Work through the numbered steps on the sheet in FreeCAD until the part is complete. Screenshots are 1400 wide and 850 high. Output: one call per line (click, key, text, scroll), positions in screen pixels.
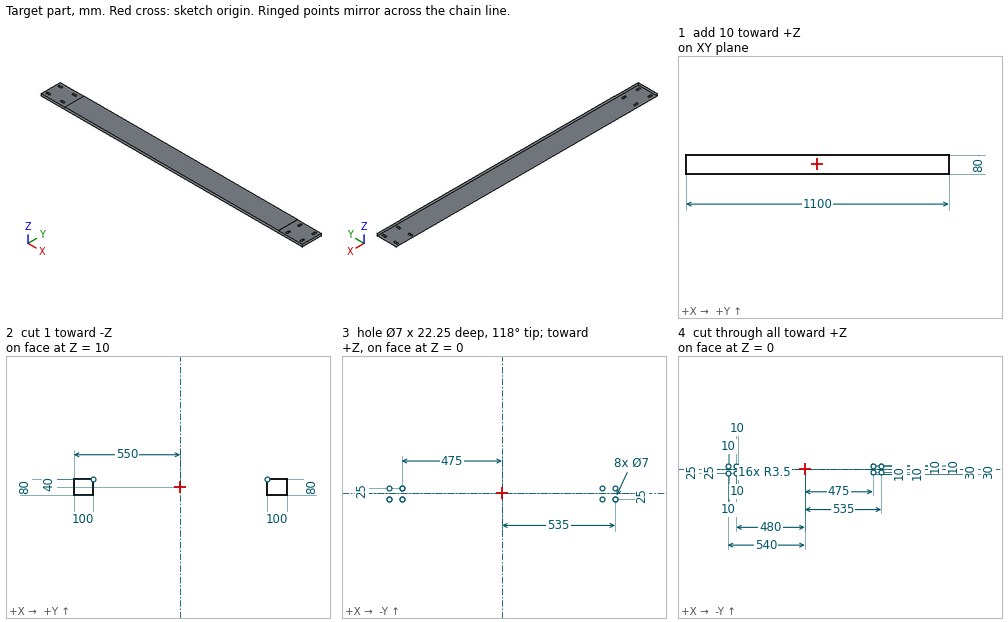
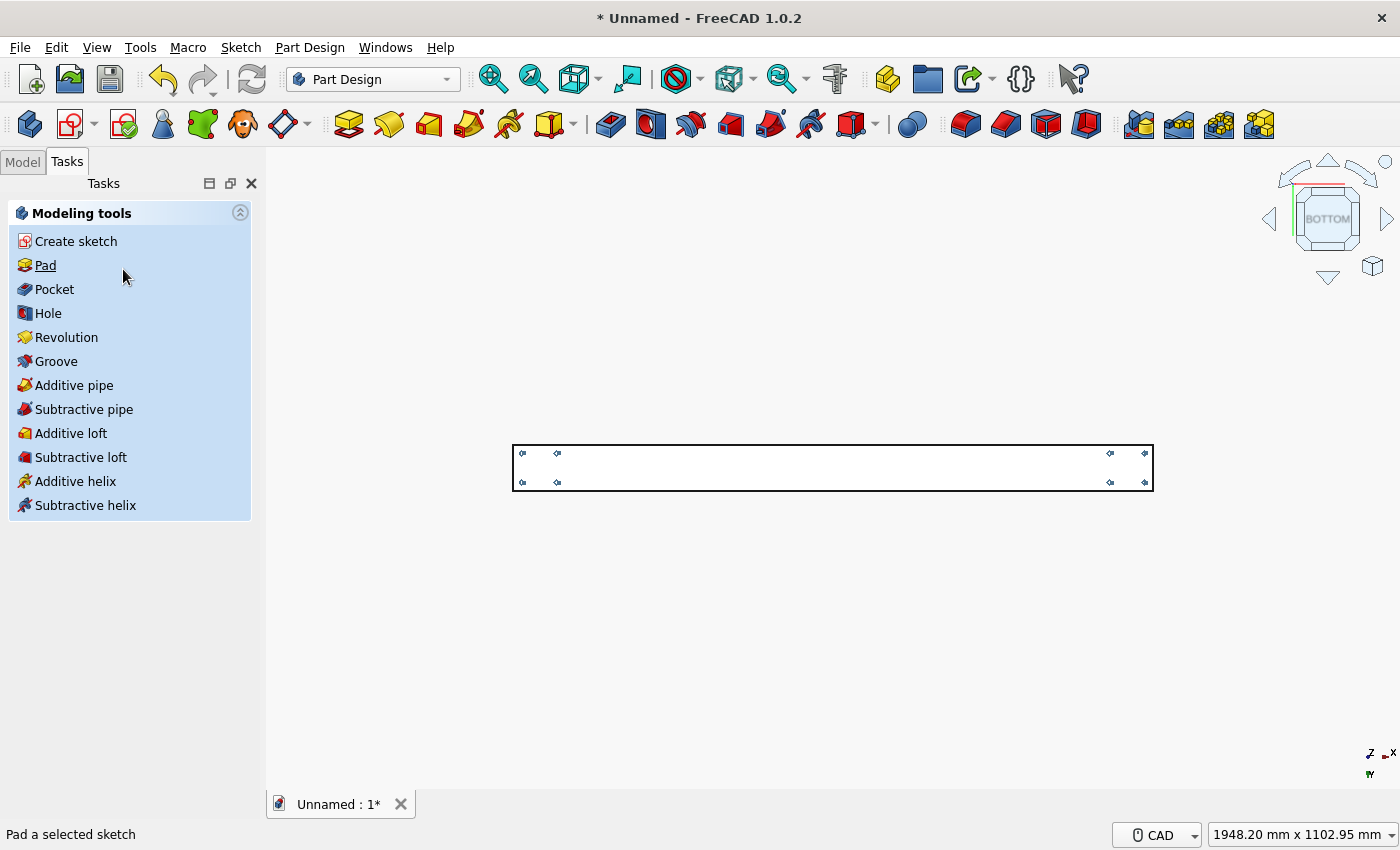
click(652, 124)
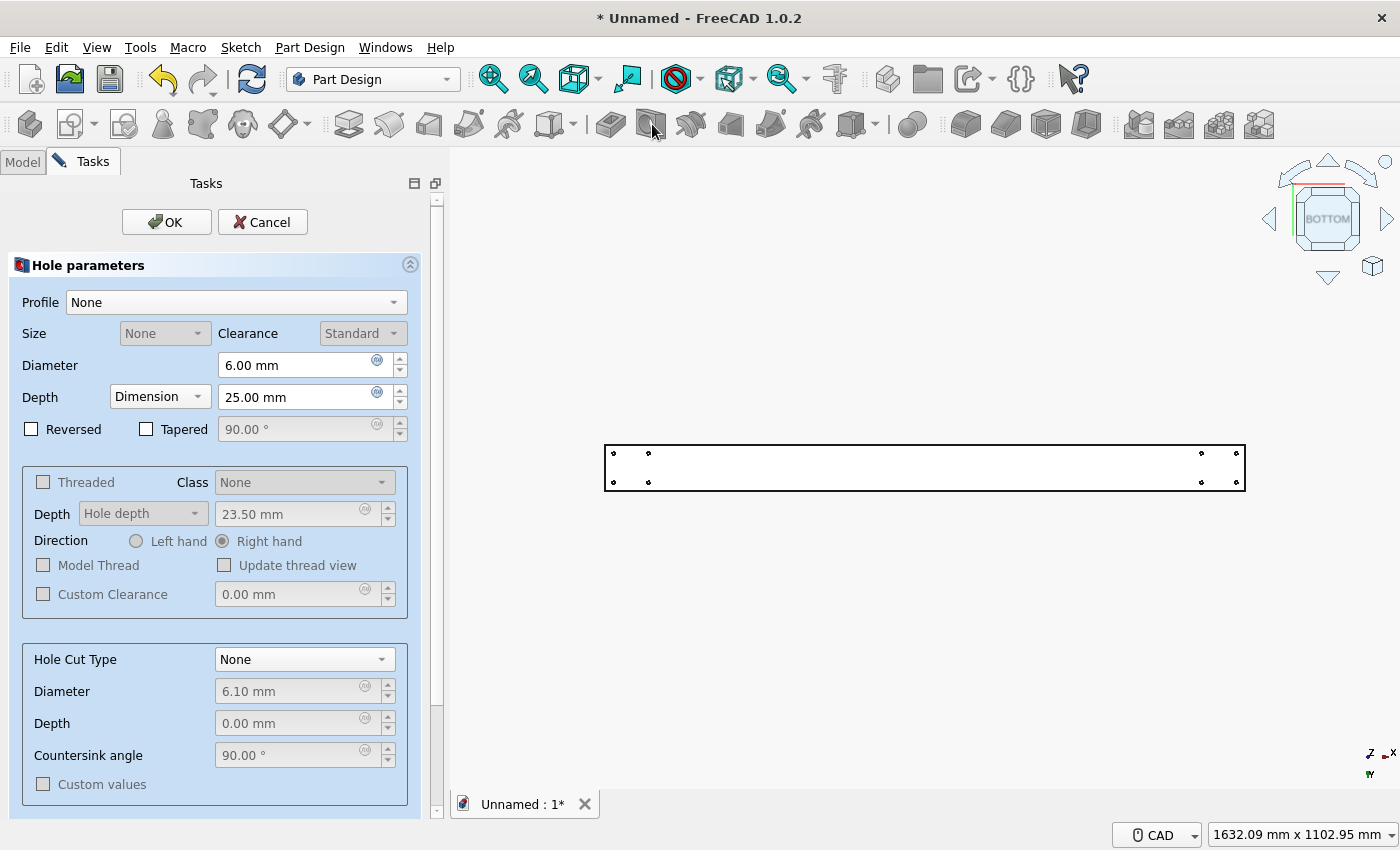
triple_click(305, 365)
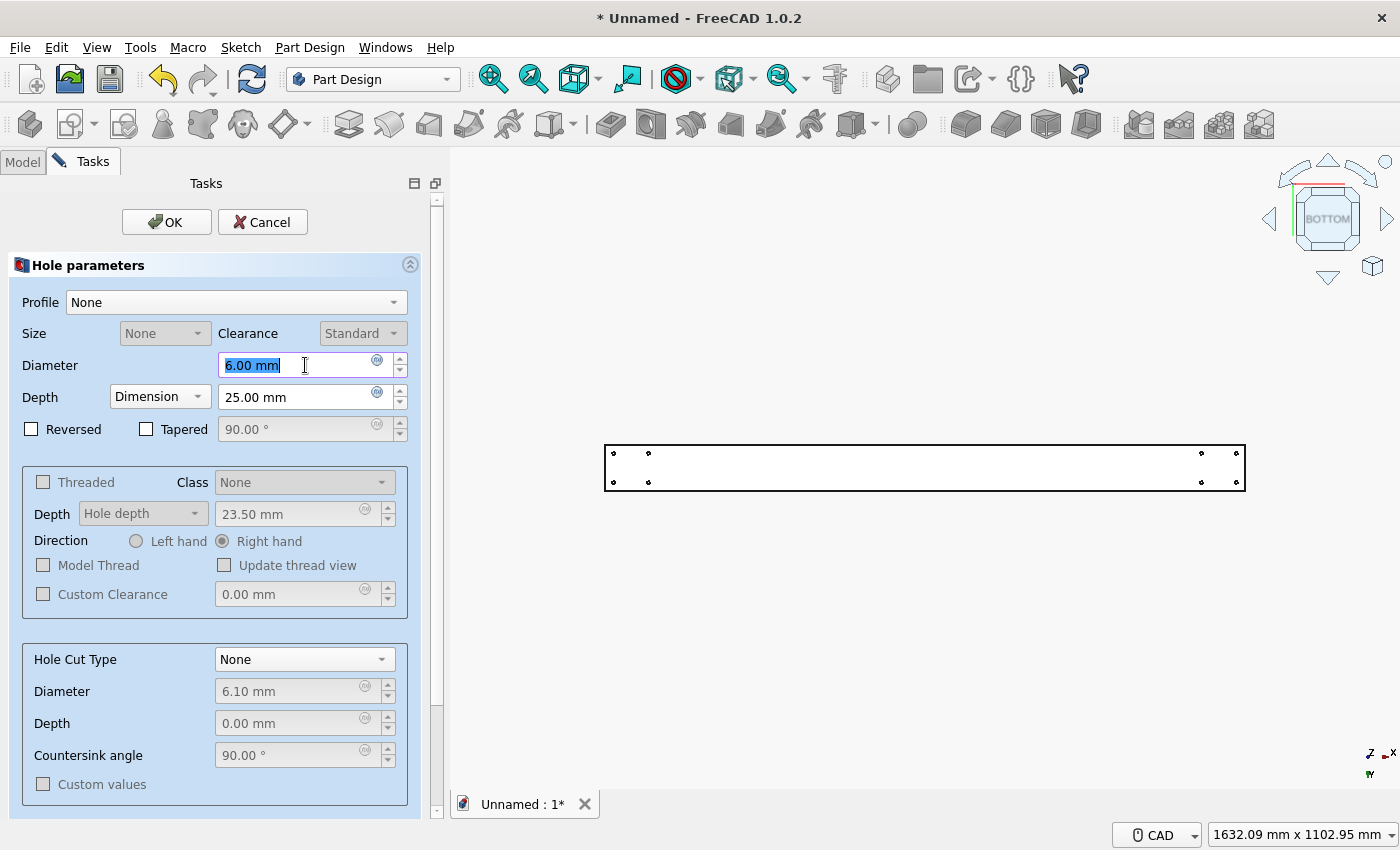
text(7)
key(Tab)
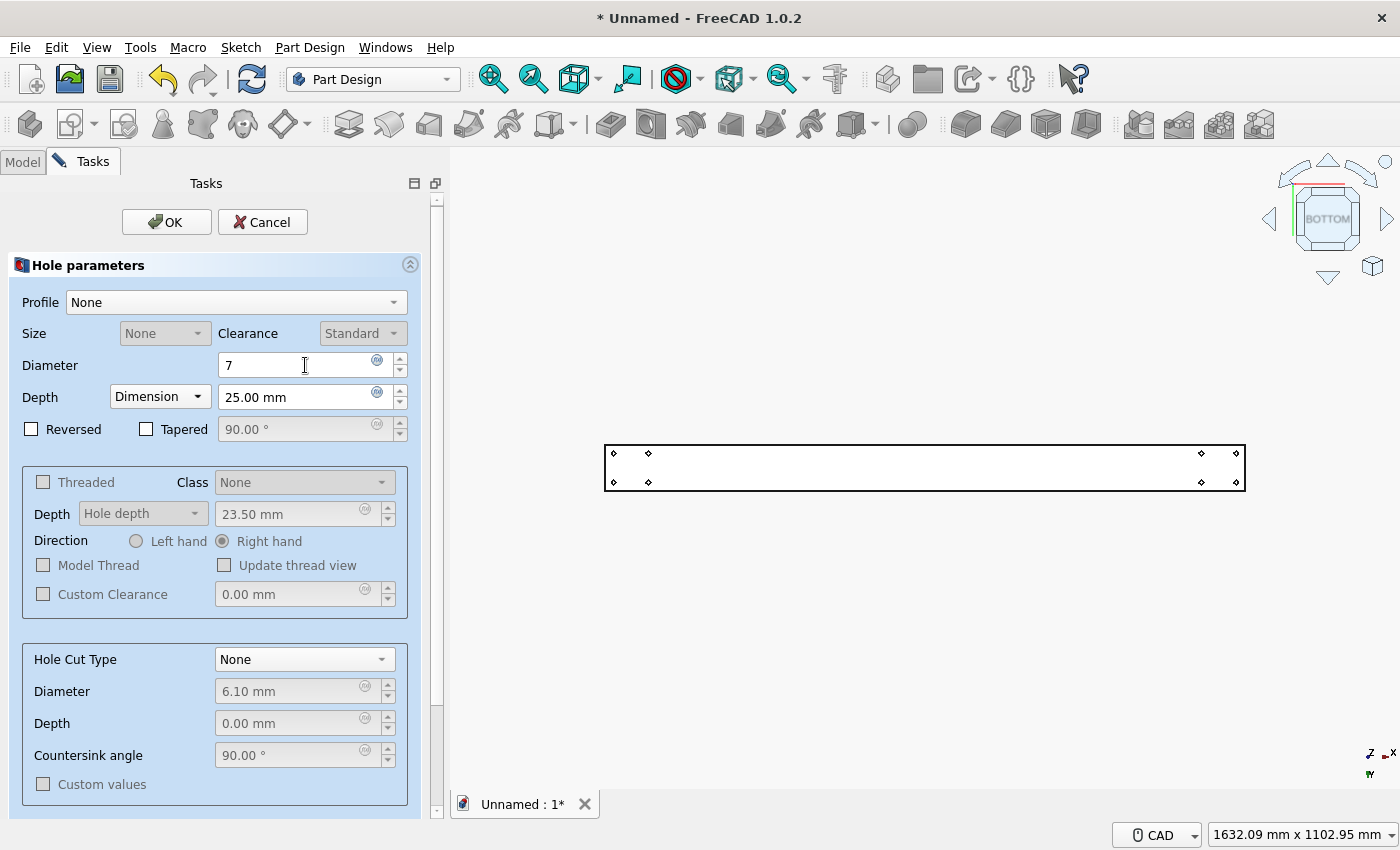
triple_click(305, 397)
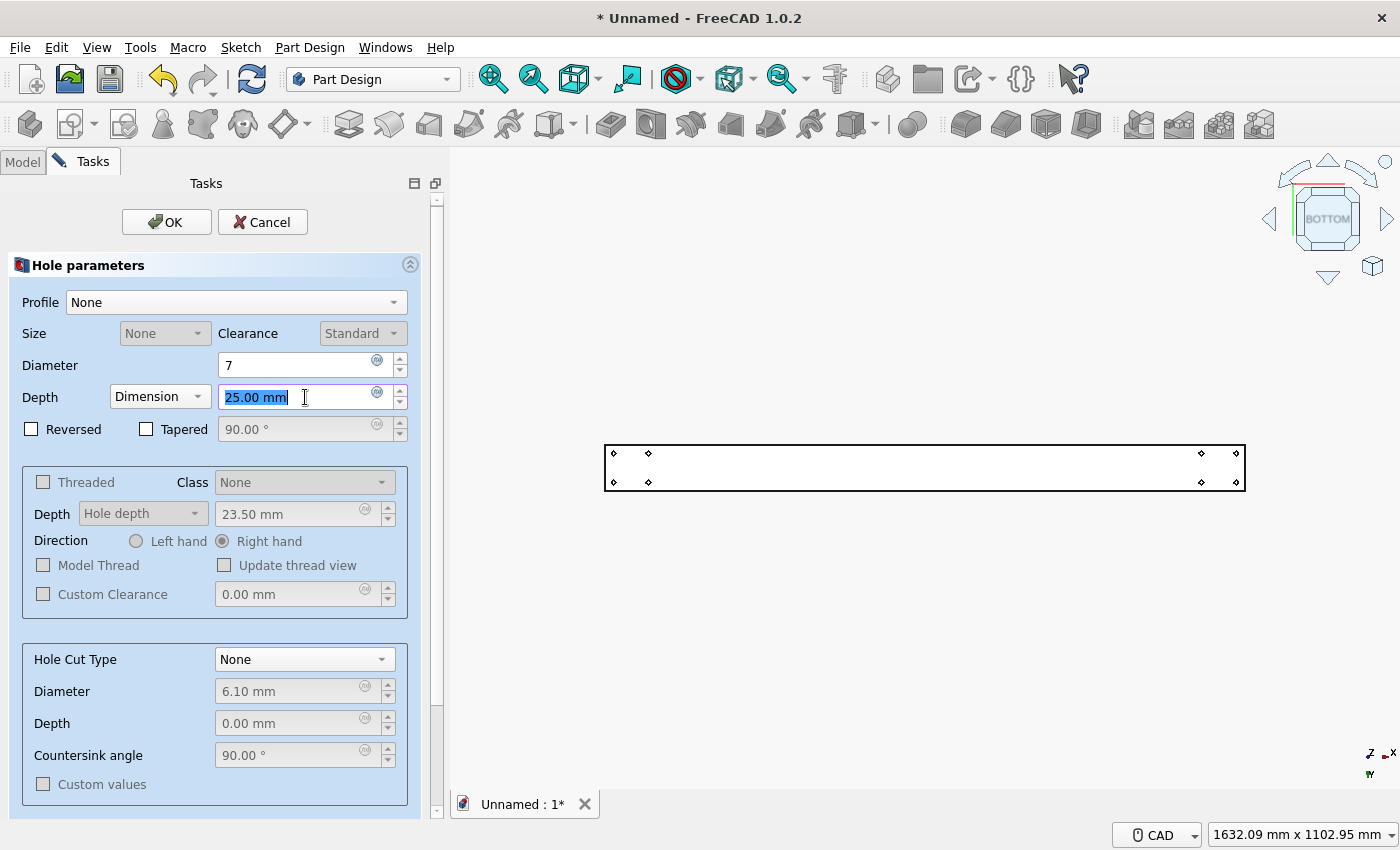
text(22.25)
key(Tab)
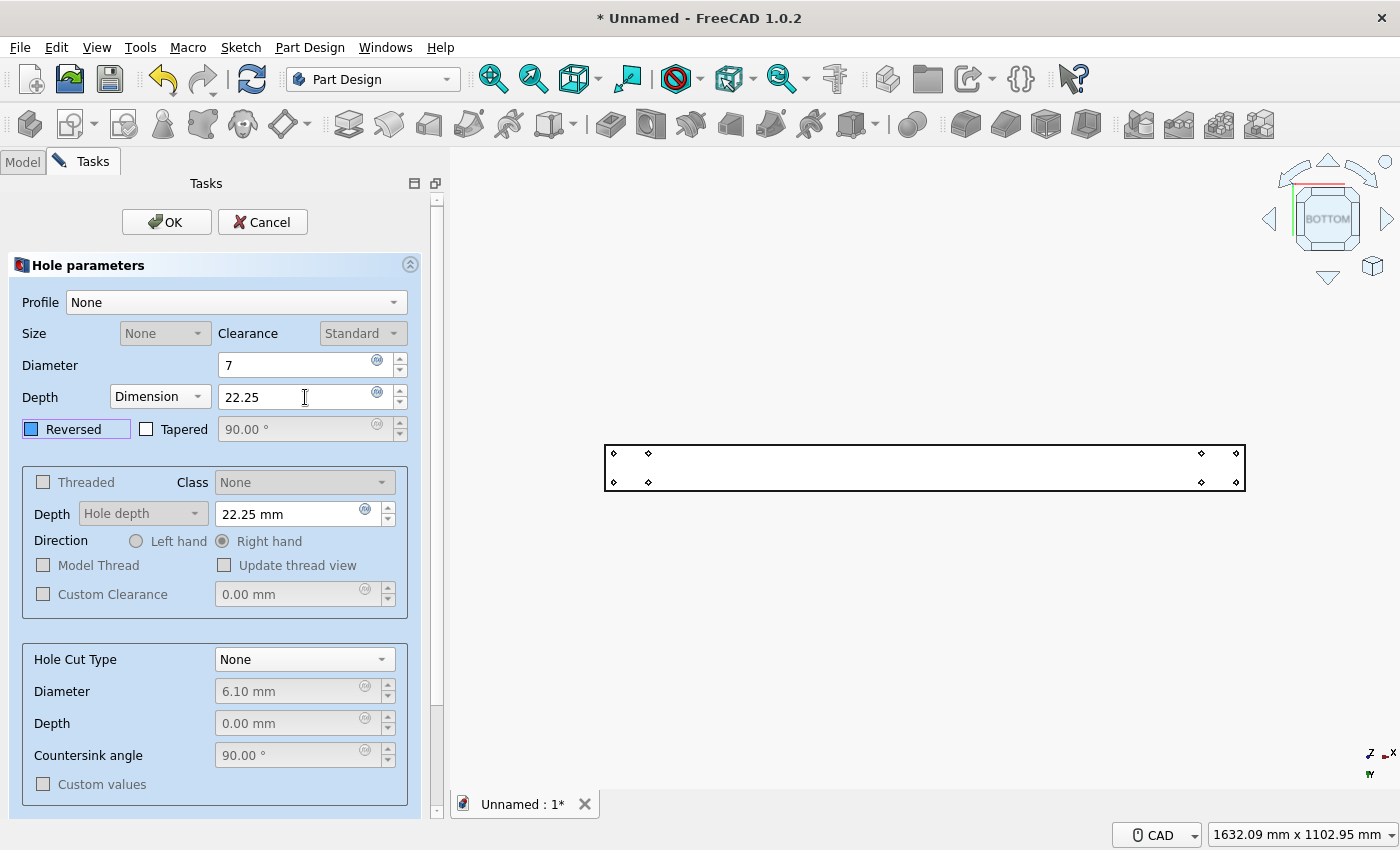
click(167, 222)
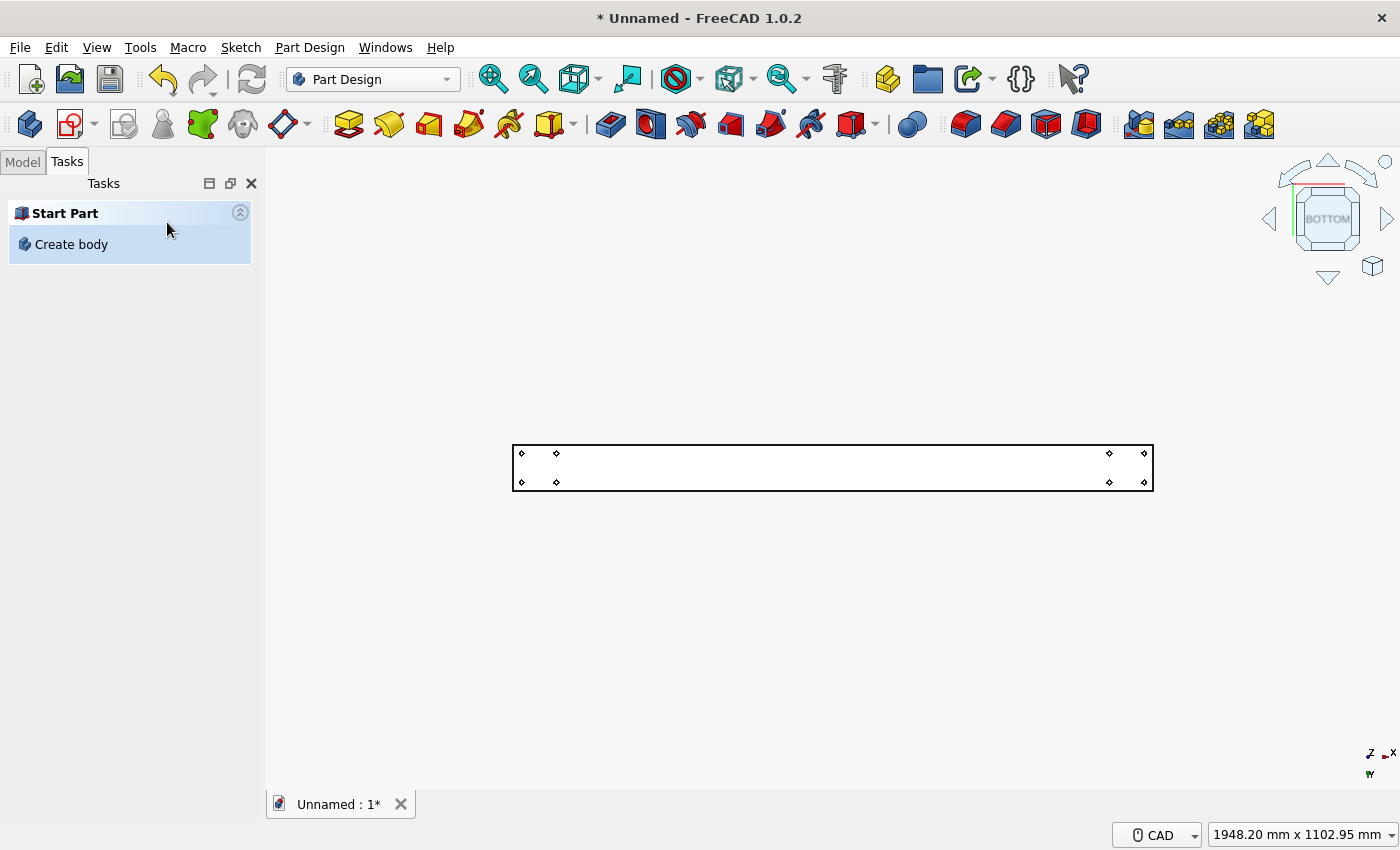
click(1016, 467)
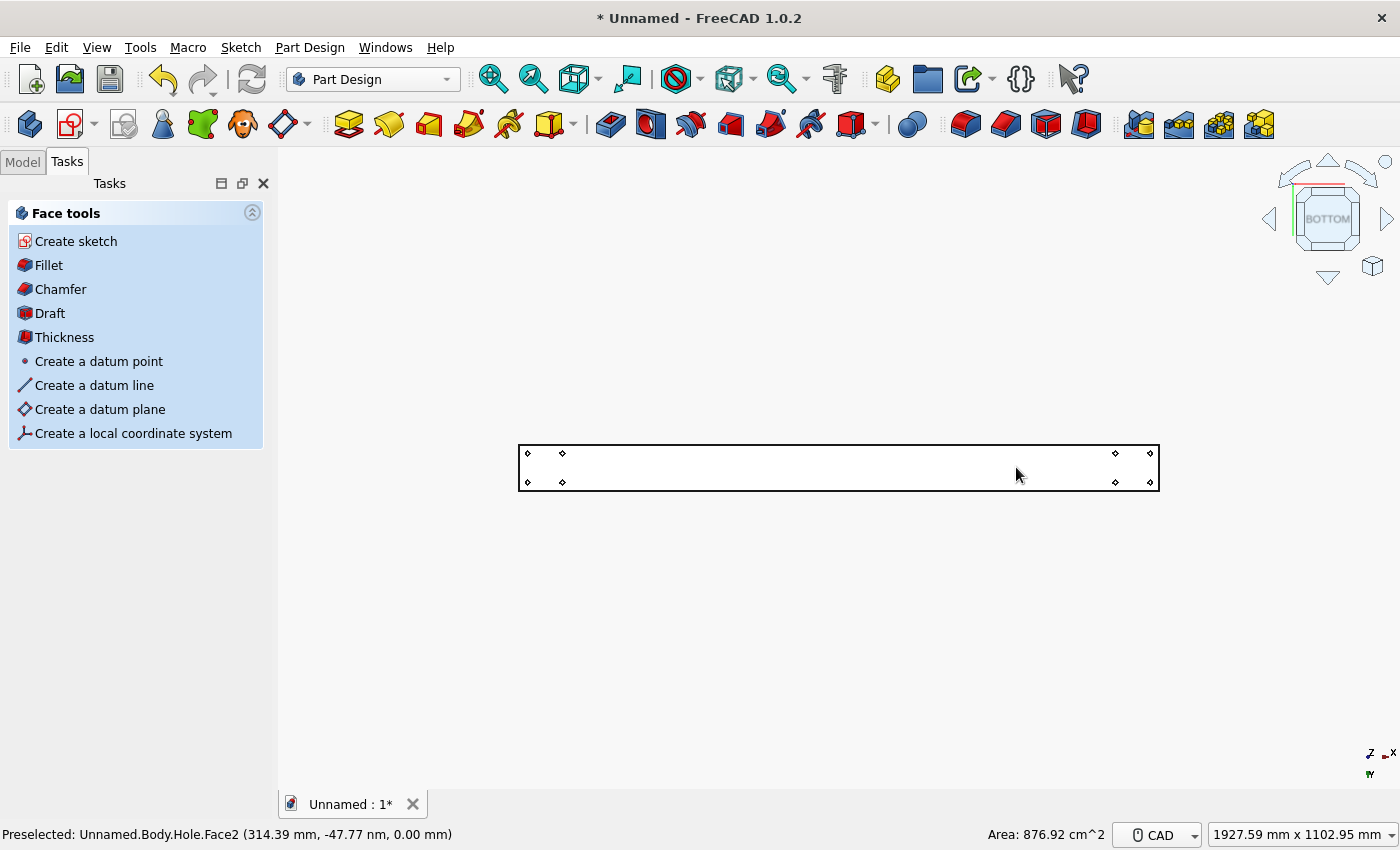
click(70, 124)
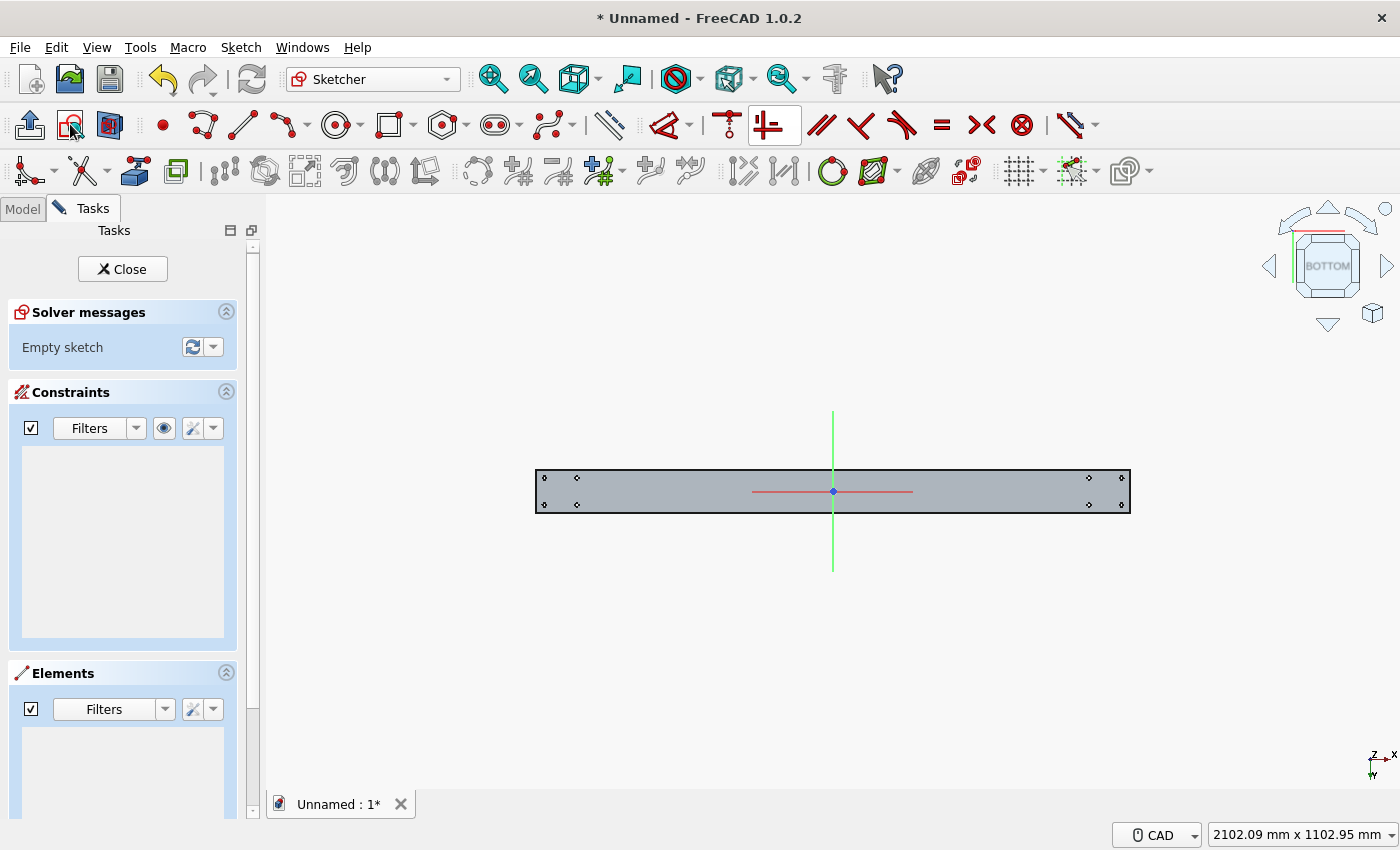
key(g)
key(s)